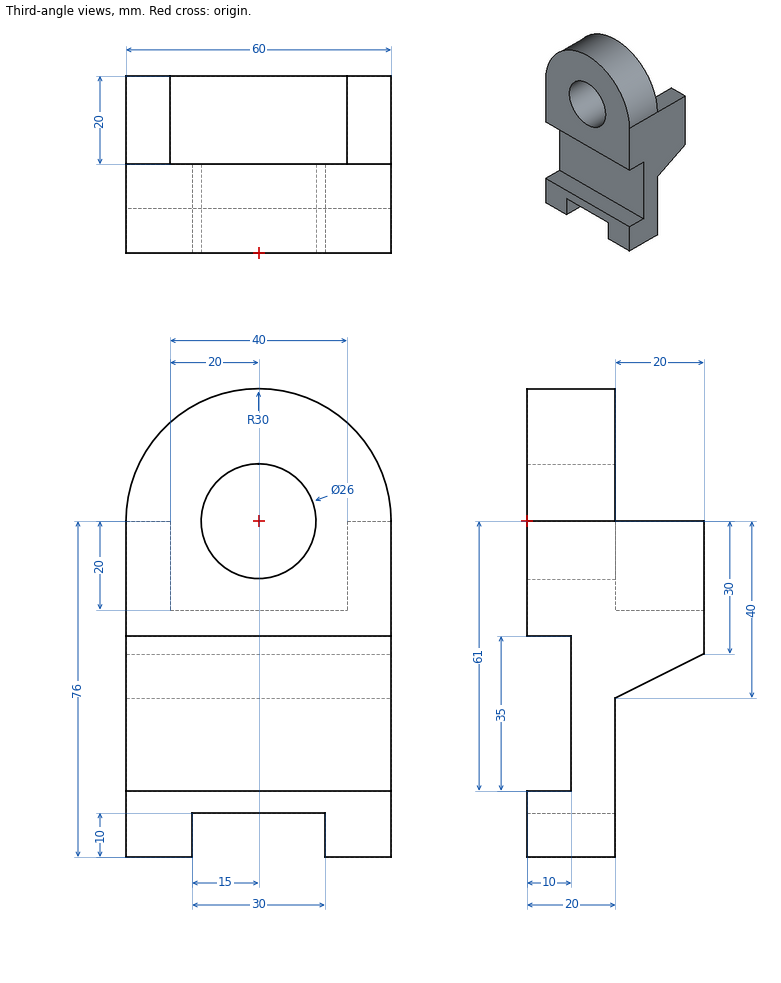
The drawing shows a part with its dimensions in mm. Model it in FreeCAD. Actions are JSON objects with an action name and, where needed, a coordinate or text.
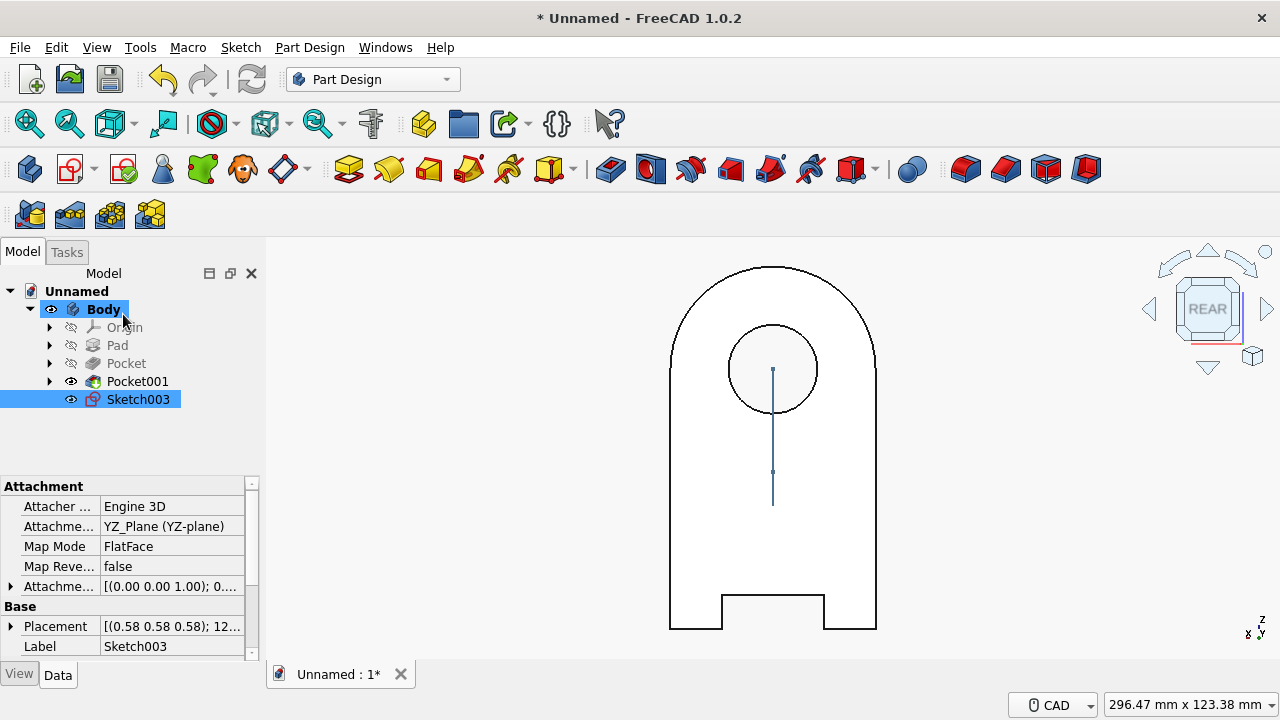
{"action": "left_click", "coordinate": [350, 170]}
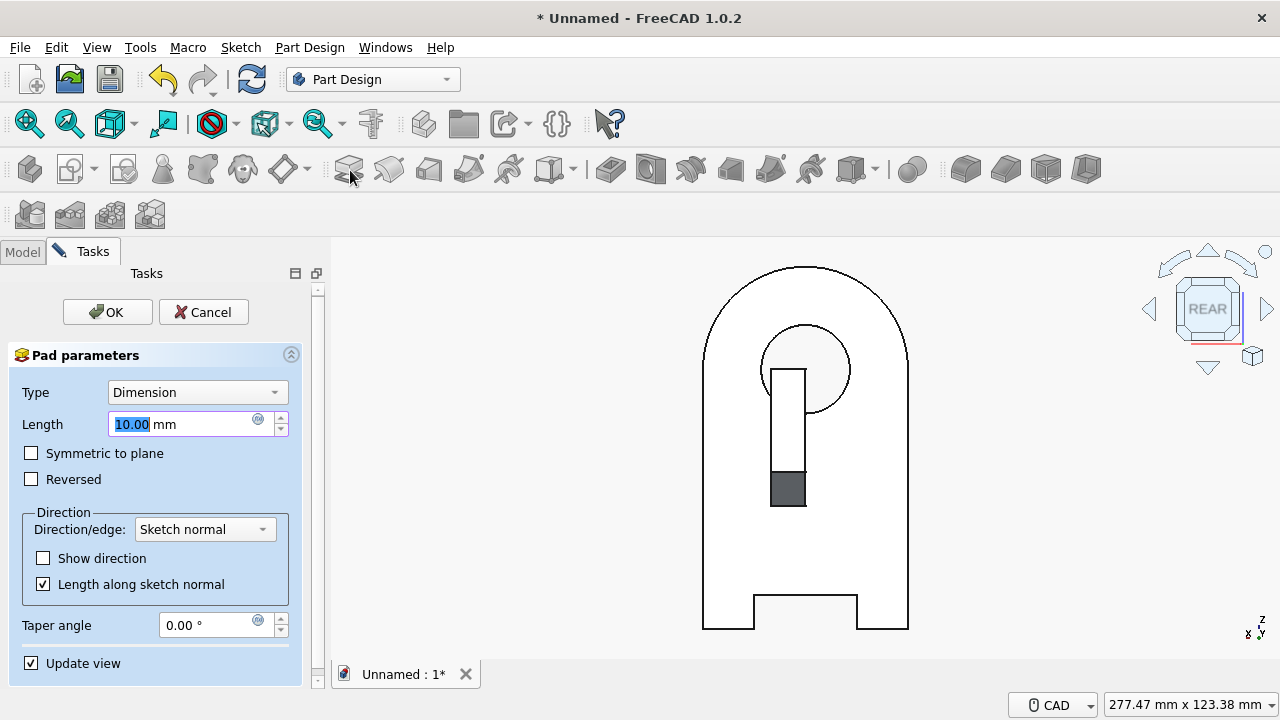
{"action": "type", "text": "60"}
{"action": "key", "text": "Tab"}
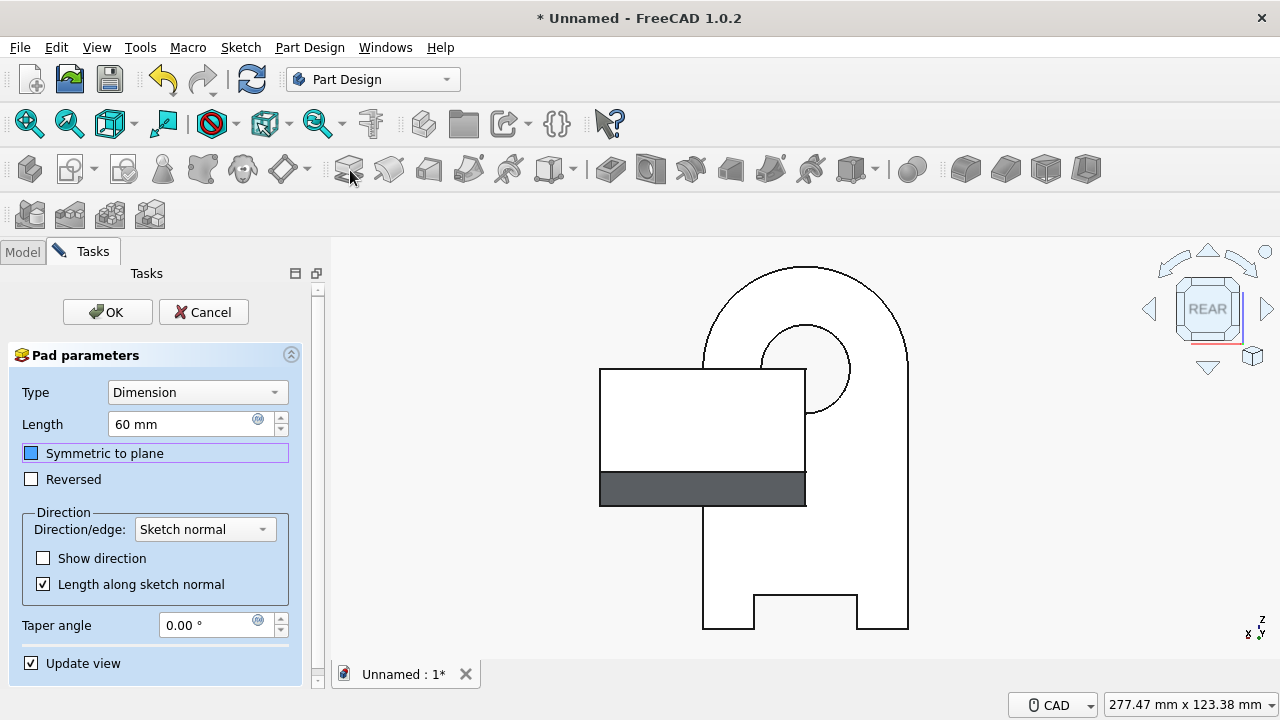
{"action": "left_click", "coordinate": [30, 453]}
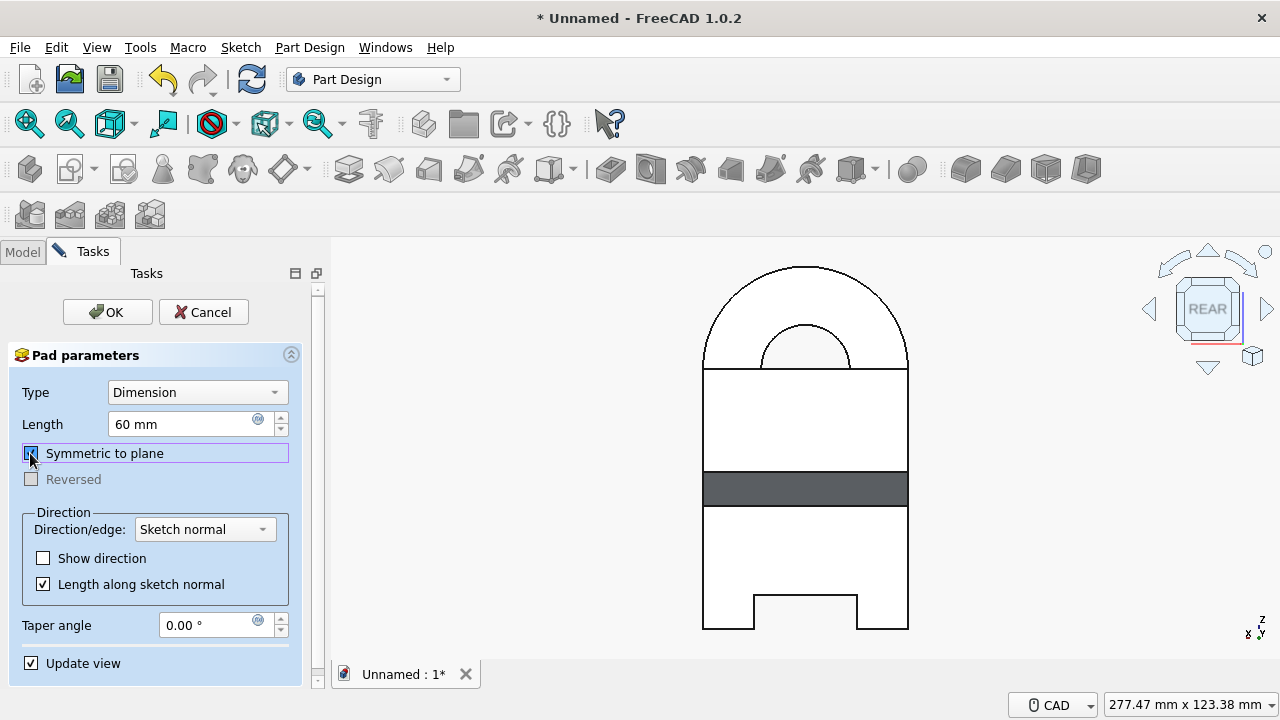
{"action": "left_click", "coordinate": [108, 312]}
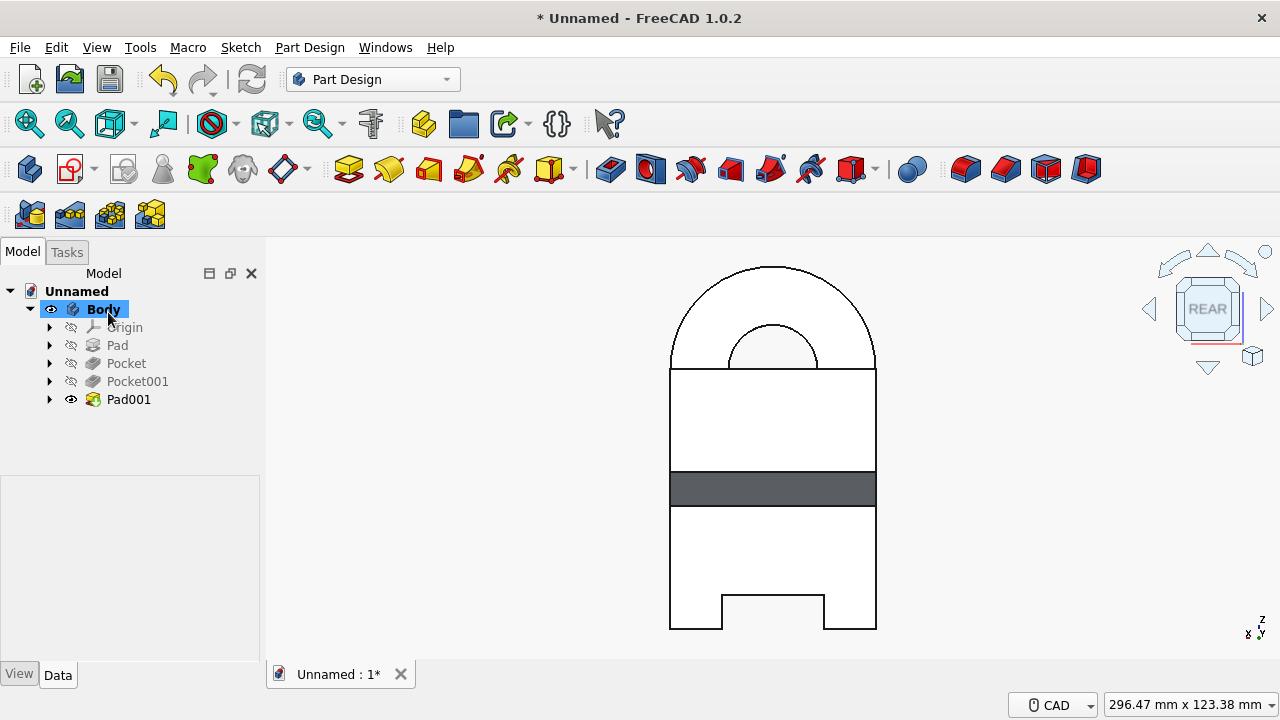
{"action": "left_click", "coordinate": [744, 420]}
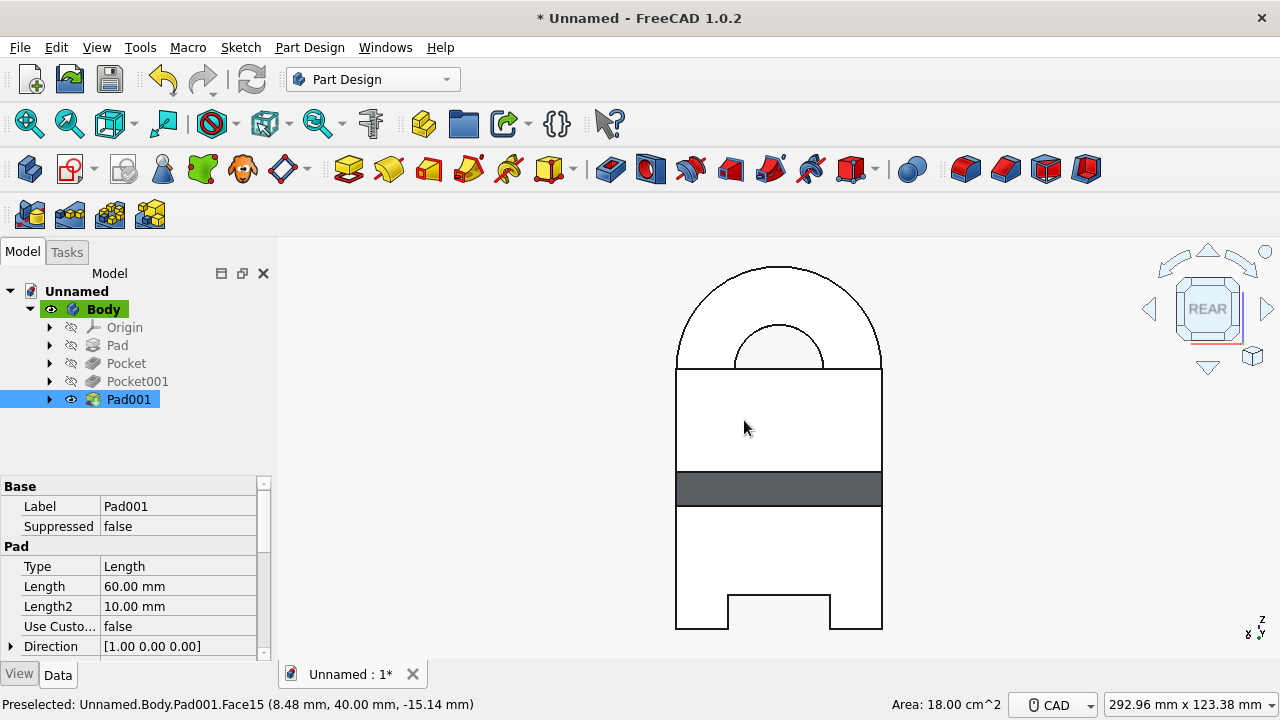
{"action": "left_click", "coordinate": [70, 170]}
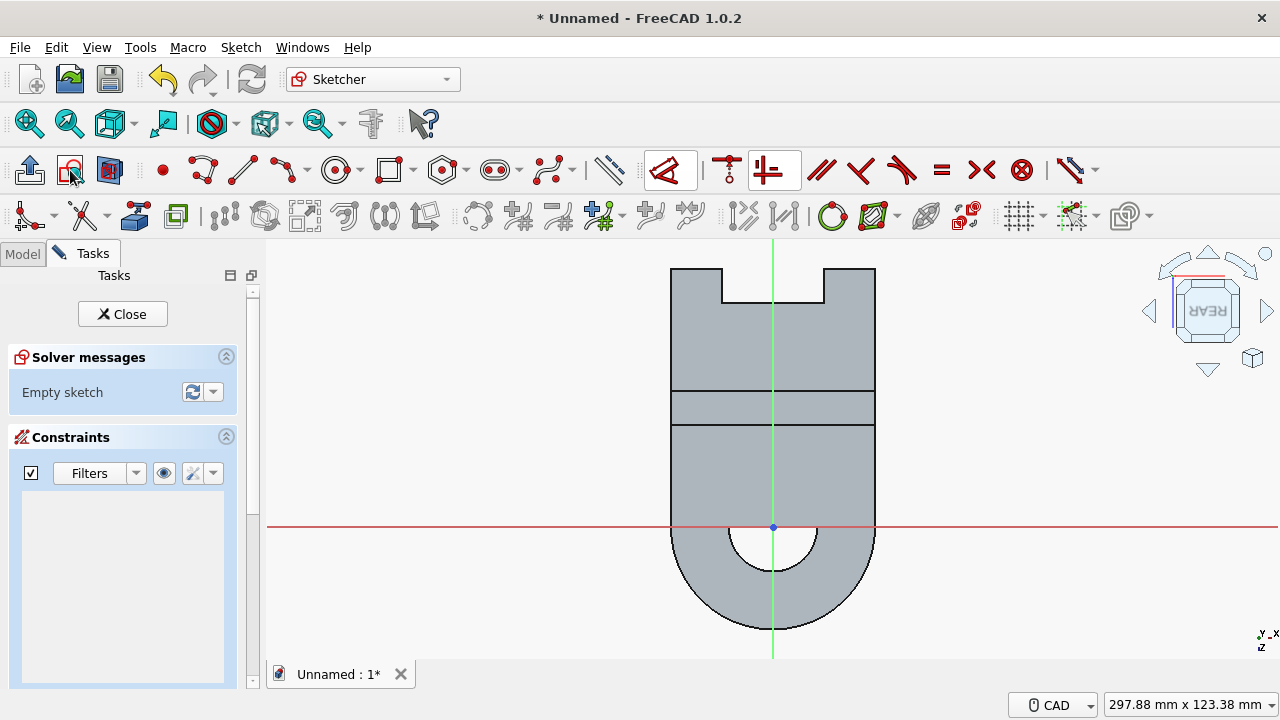
{"action": "scroll", "coordinate": [795, 508], "scroll_direction": "up", "scroll_amount": 7}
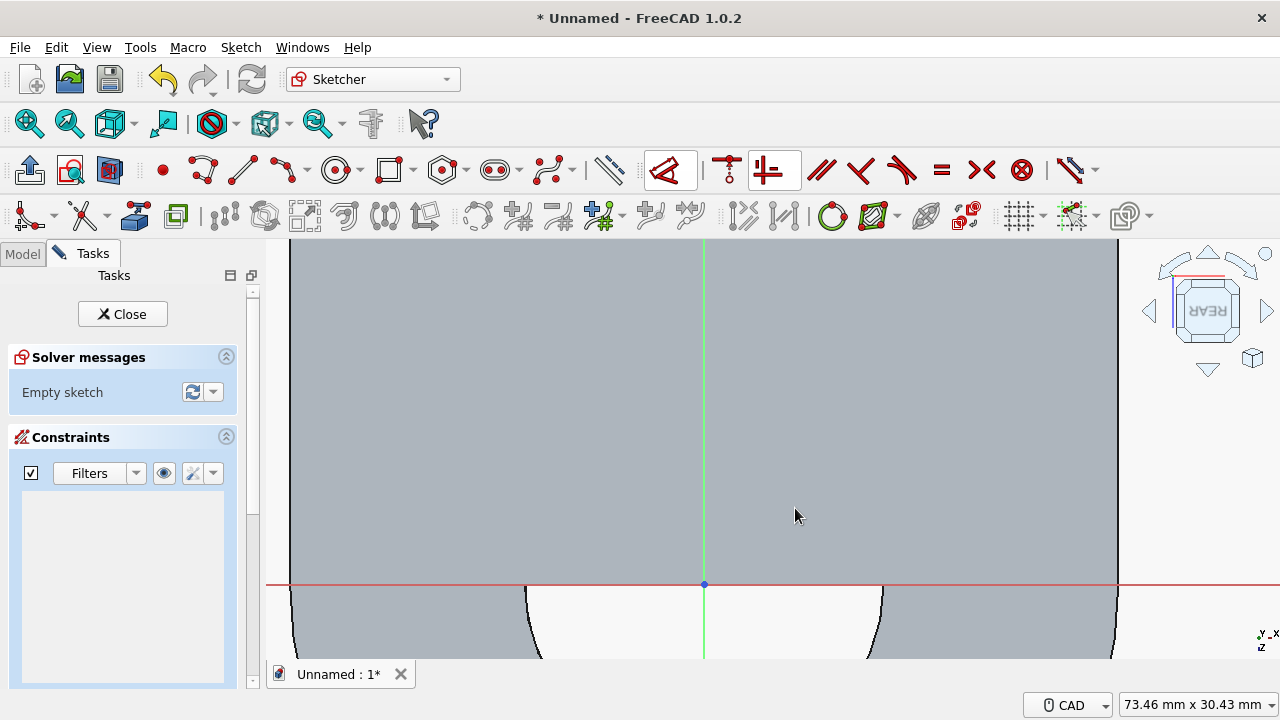
{"action": "key", "text": "g r"}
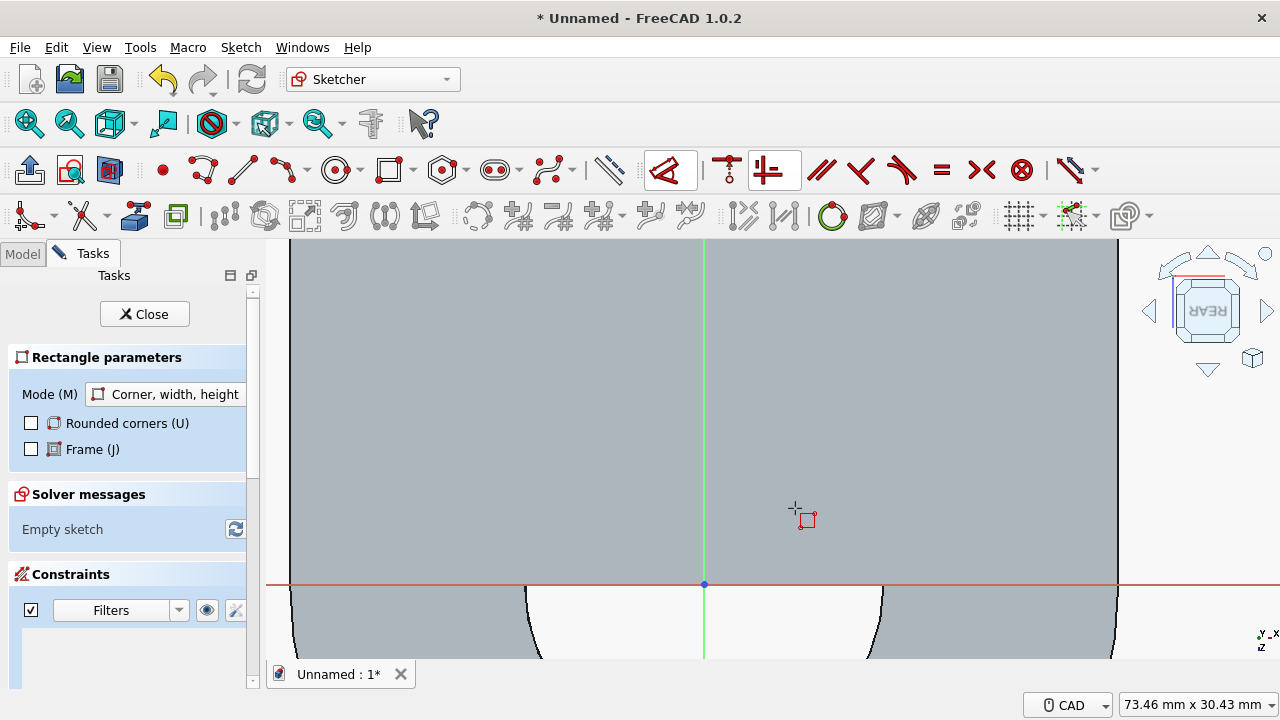
{"action": "left_click", "coordinate": [428, 309]}
{"action": "left_click", "coordinate": [980, 585]}
{"action": "key", "text": "Escape"}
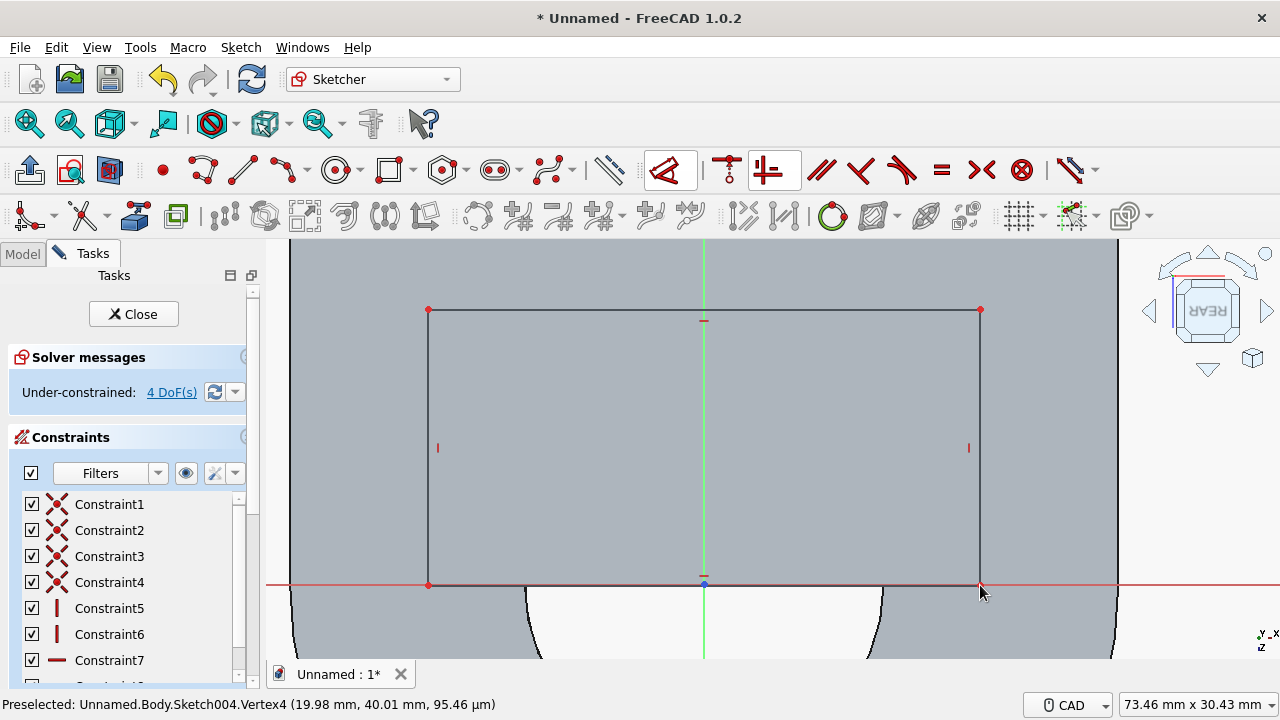
{"action": "left_click", "coordinate": [428, 586]}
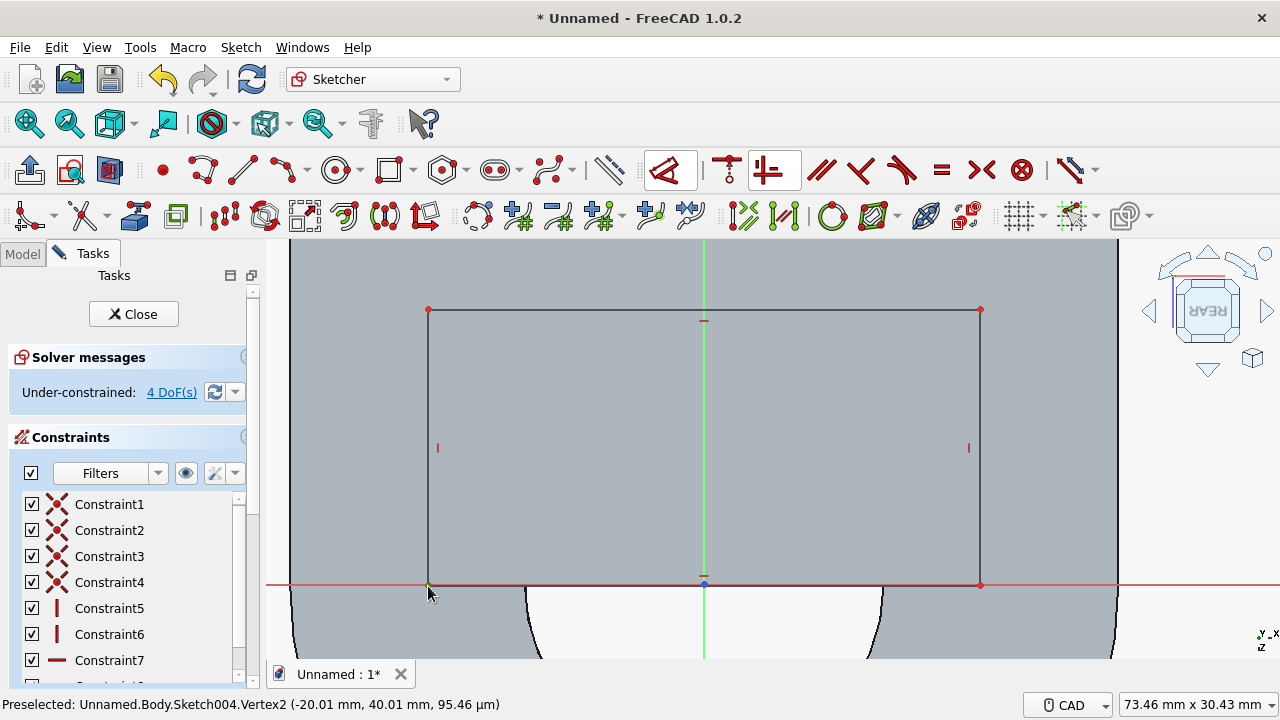
{"action": "left_click", "coordinate": [353, 585]}